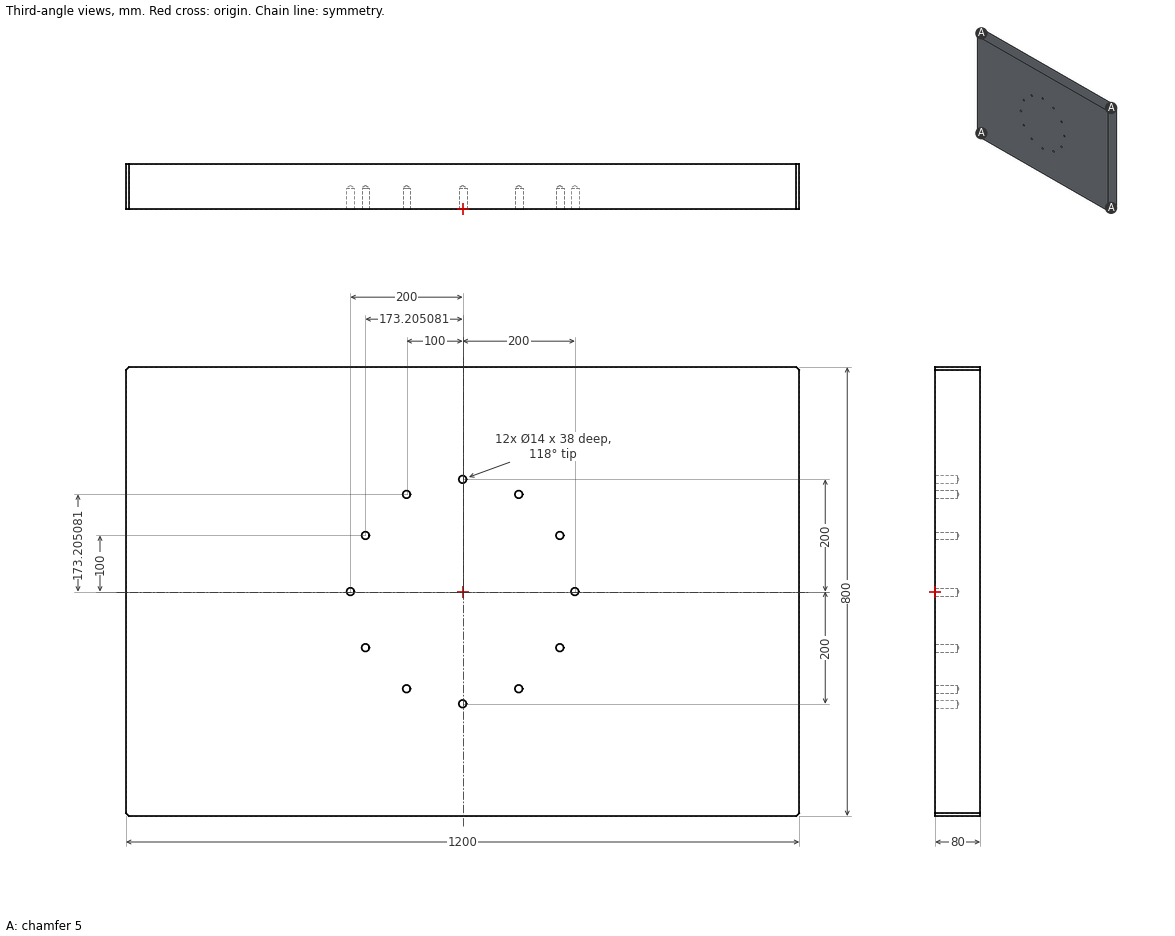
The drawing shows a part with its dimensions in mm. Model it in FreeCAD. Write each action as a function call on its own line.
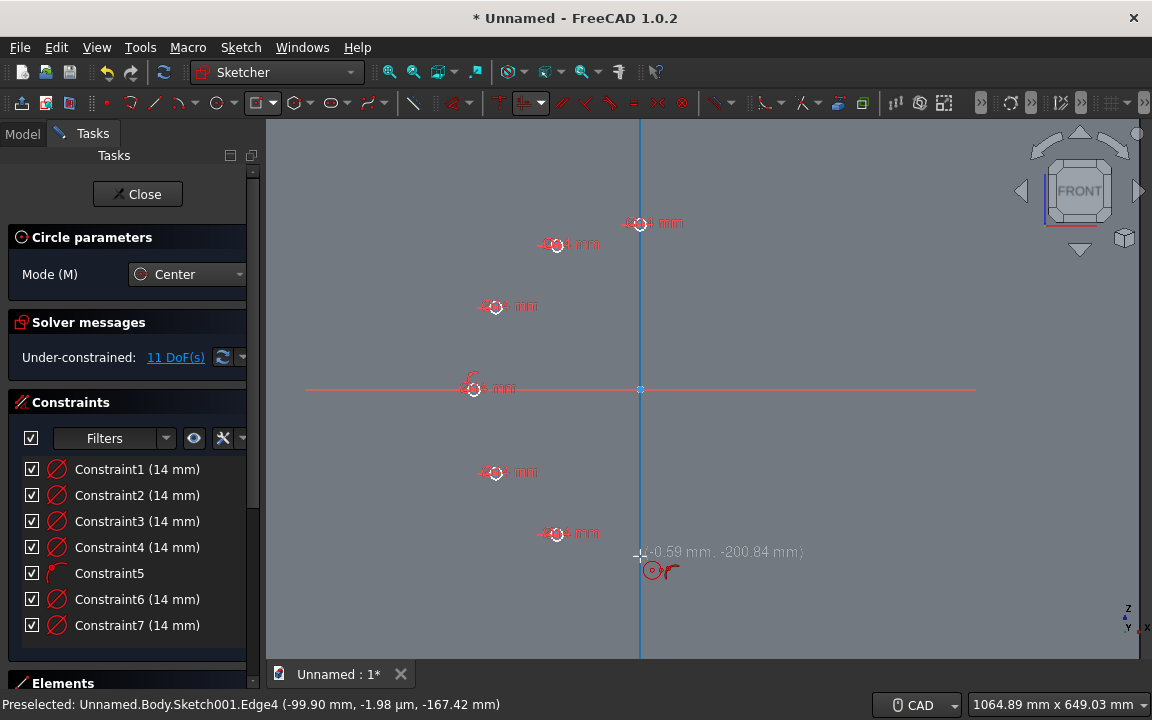
click(640, 556)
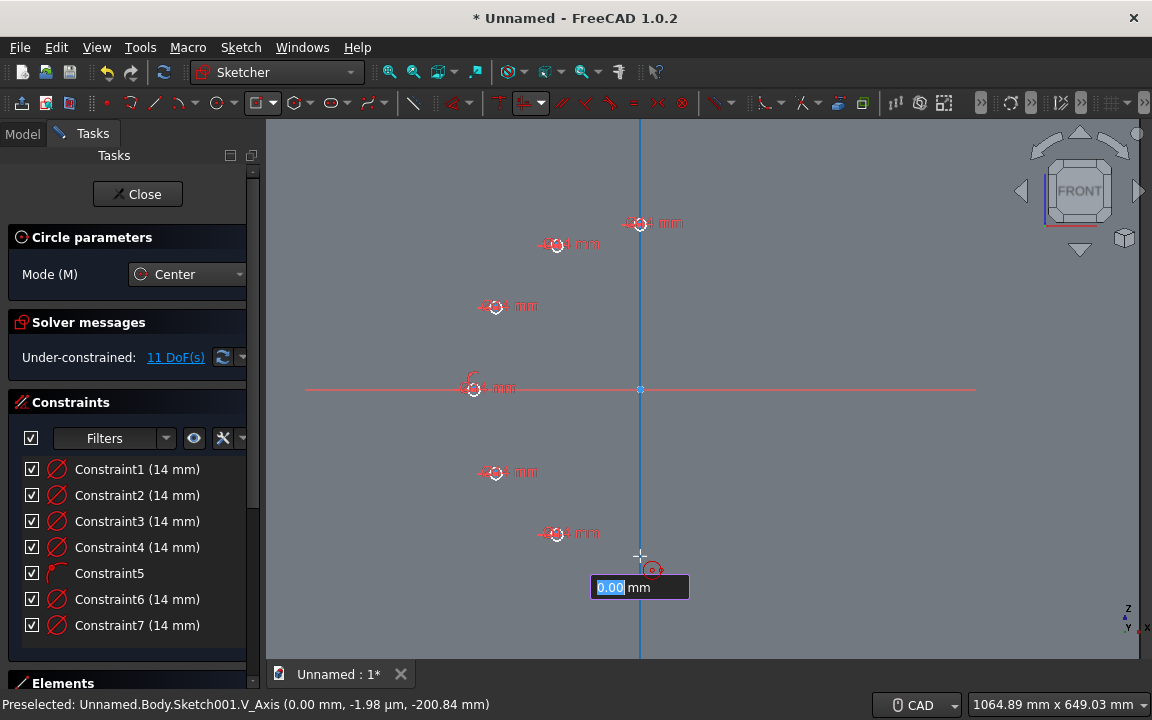
scroll(646, 554, up, 6)
move(645, 553)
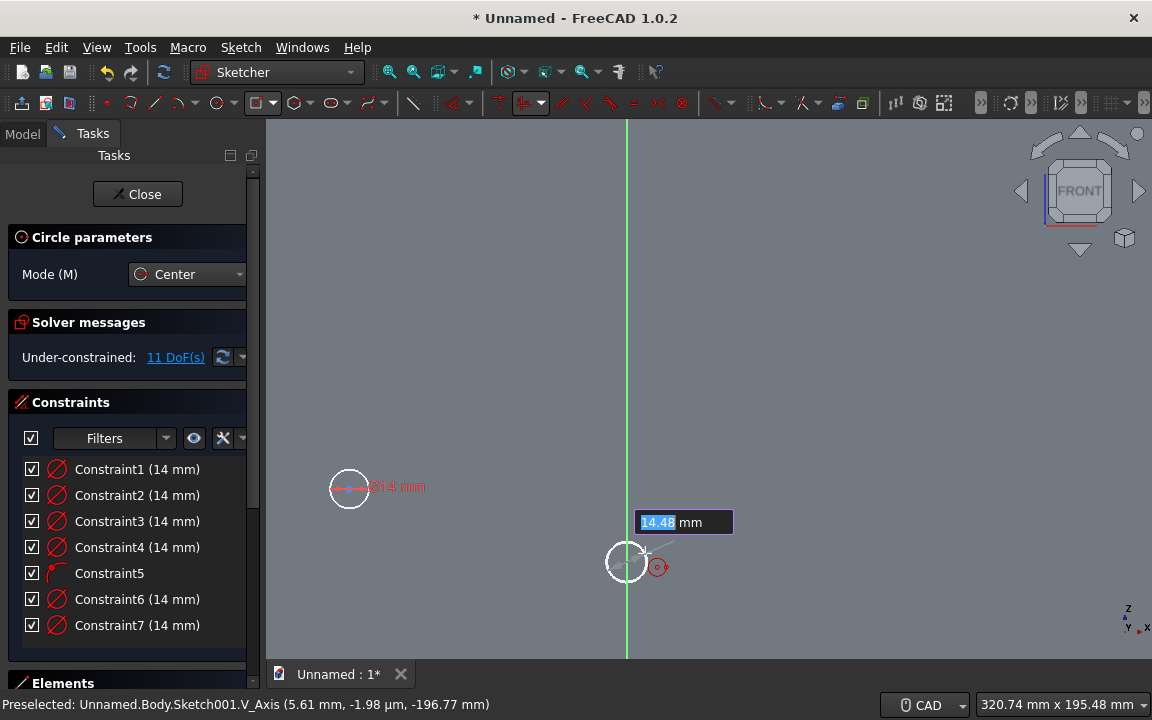
text(14)
key(Return)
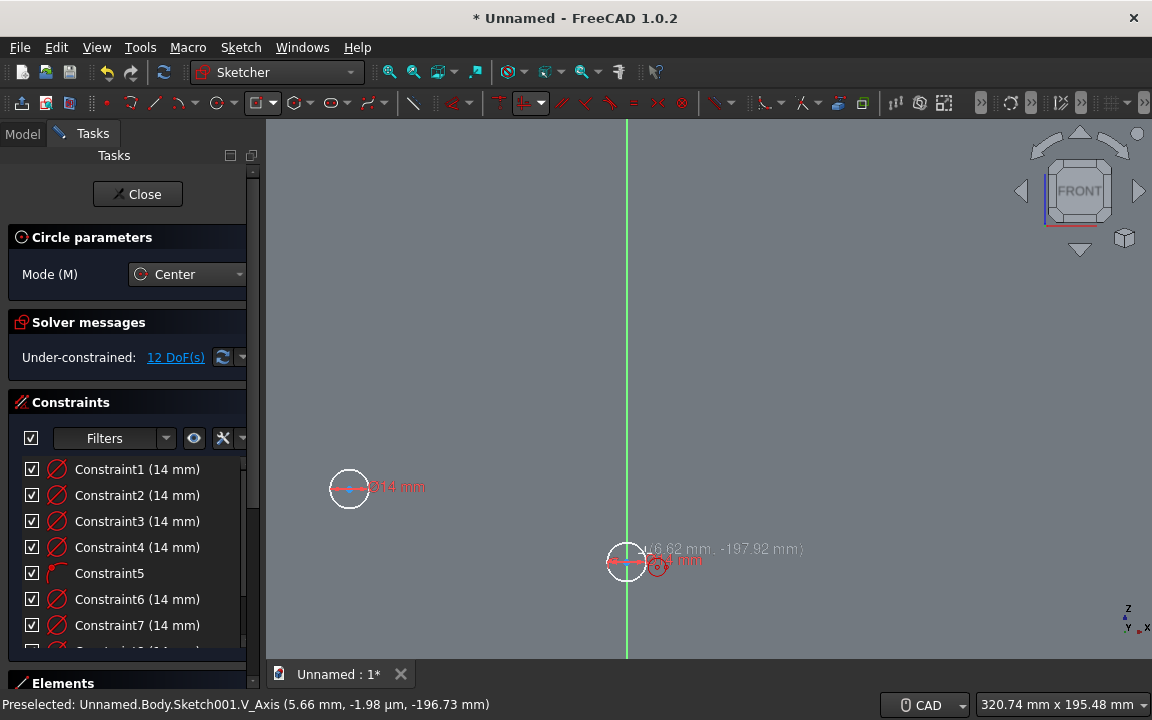
click(903, 486)
move(917, 472)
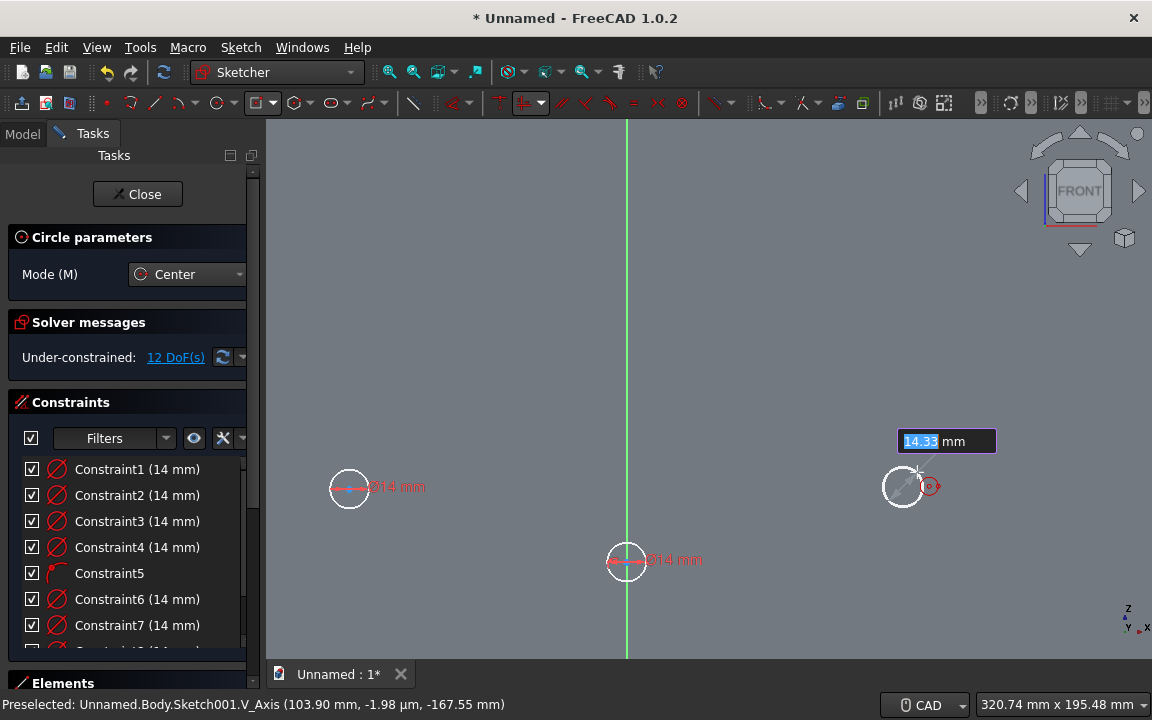
text(14)
key(Return)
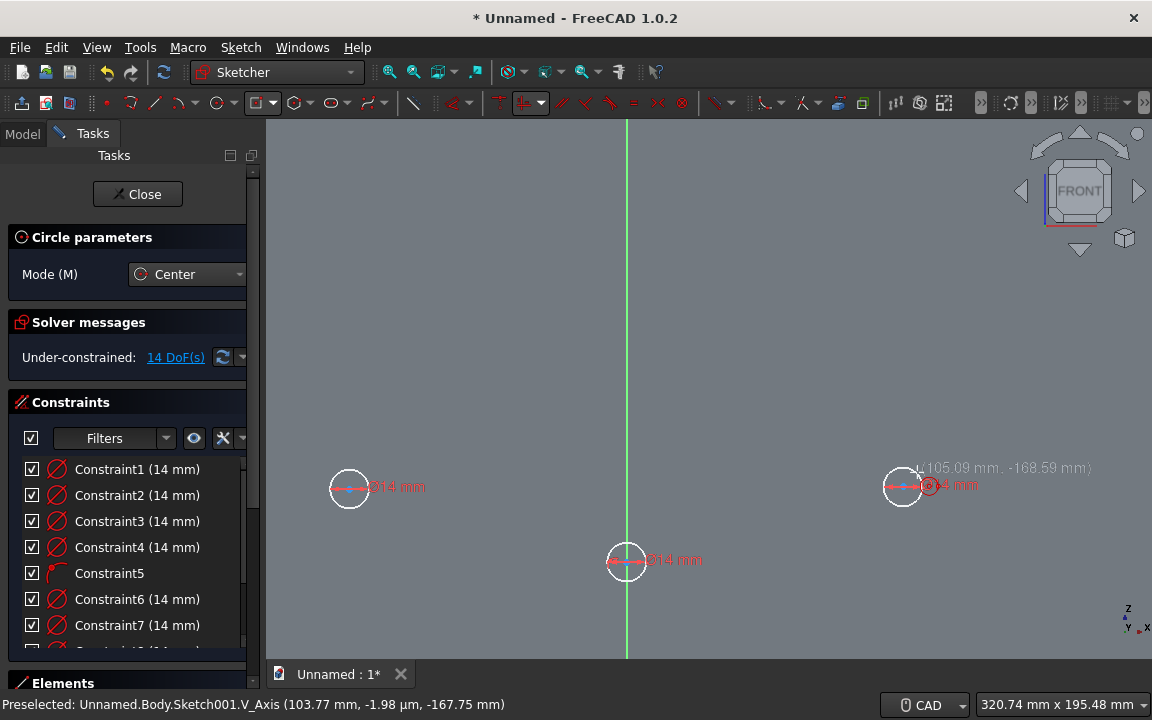
scroll(646, 554, down, 6)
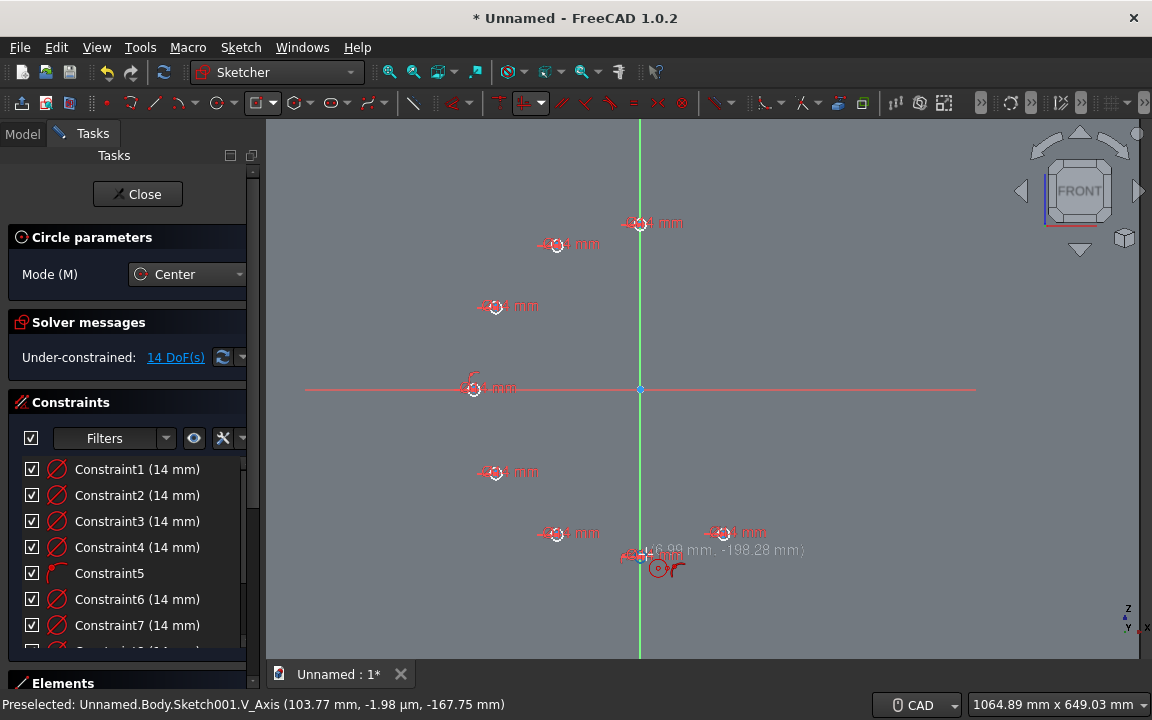
scroll(785, 473, up, 7)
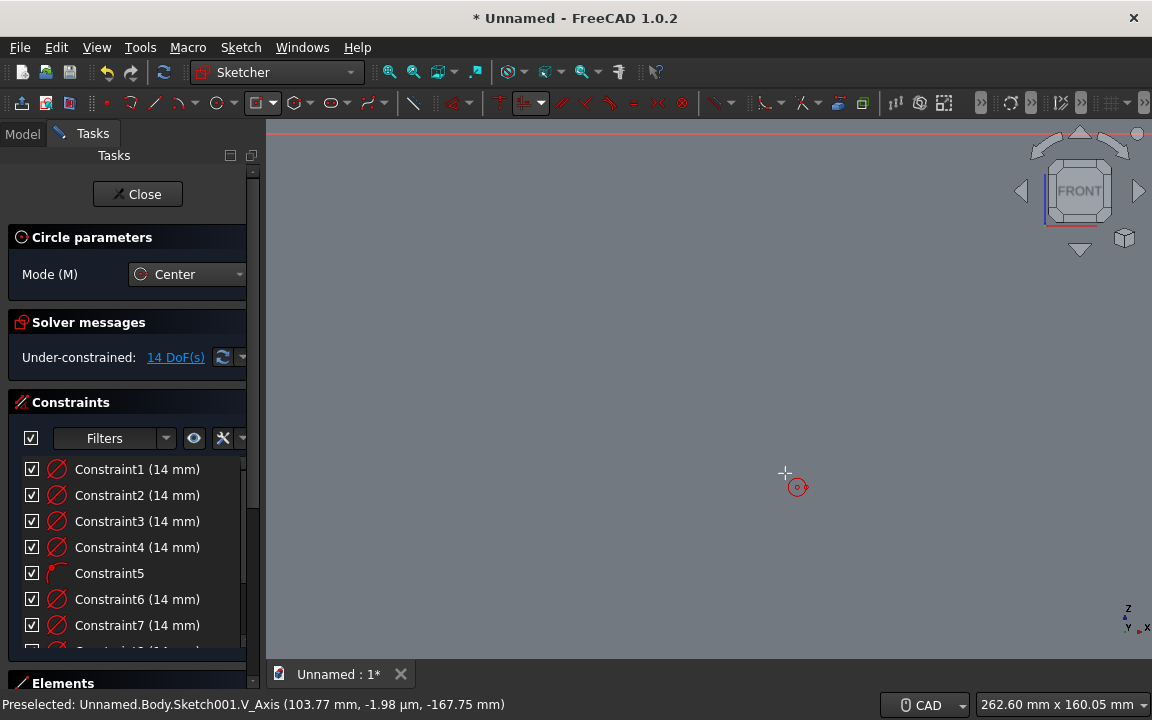
scroll(786, 472, down, 7)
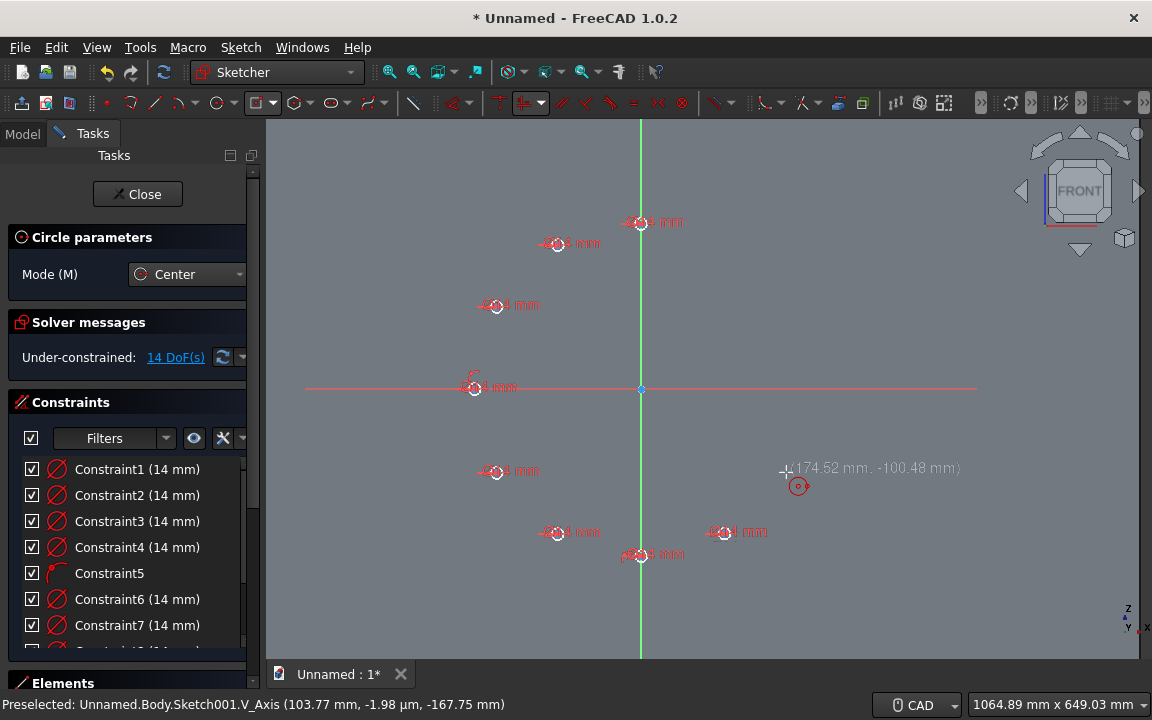
click(785, 472)
move(789, 468)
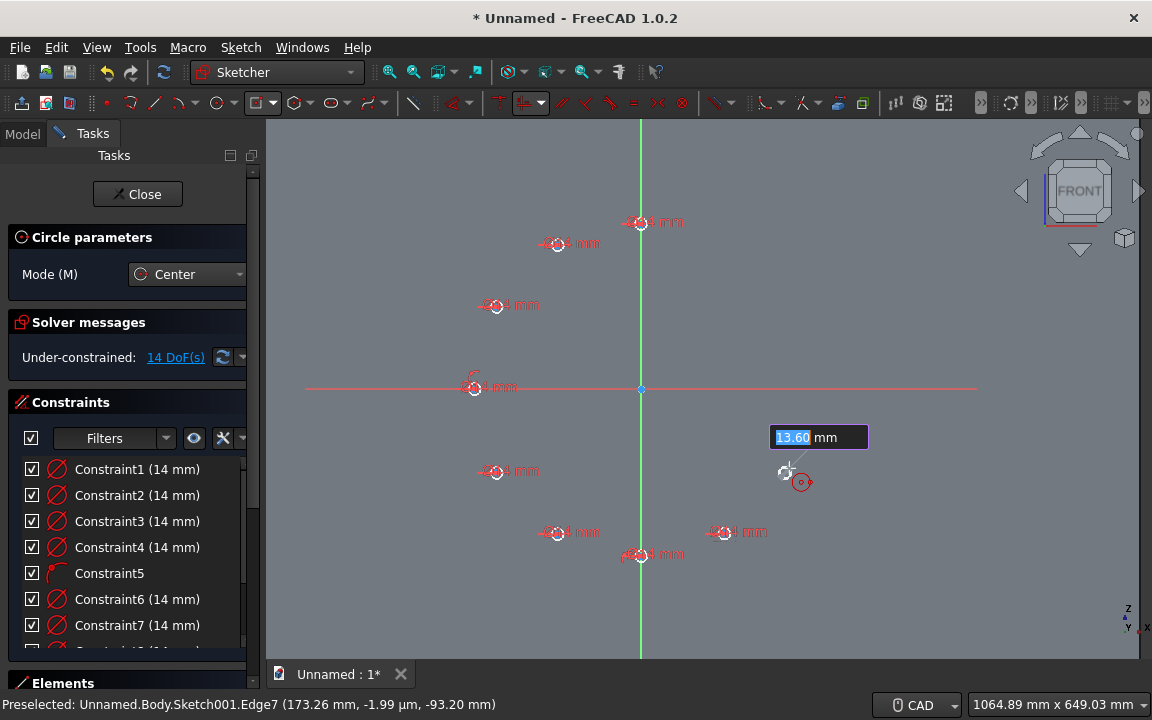
text(14)
key(Return)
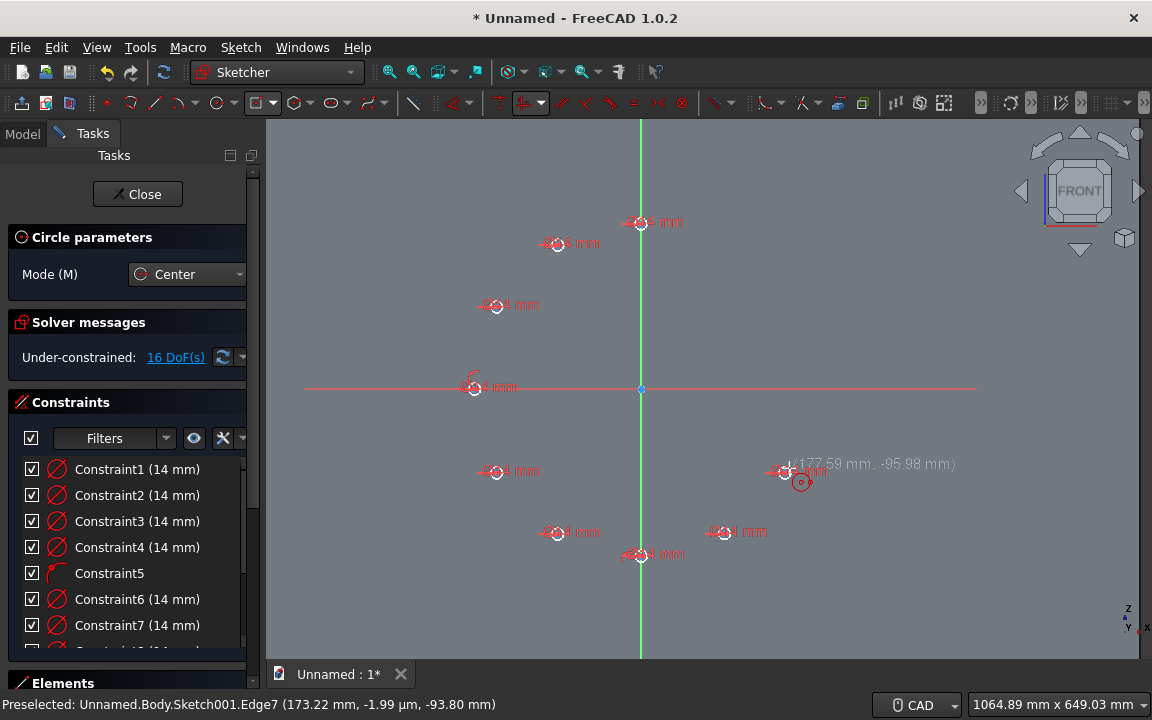
scroll(808, 389, up, 7)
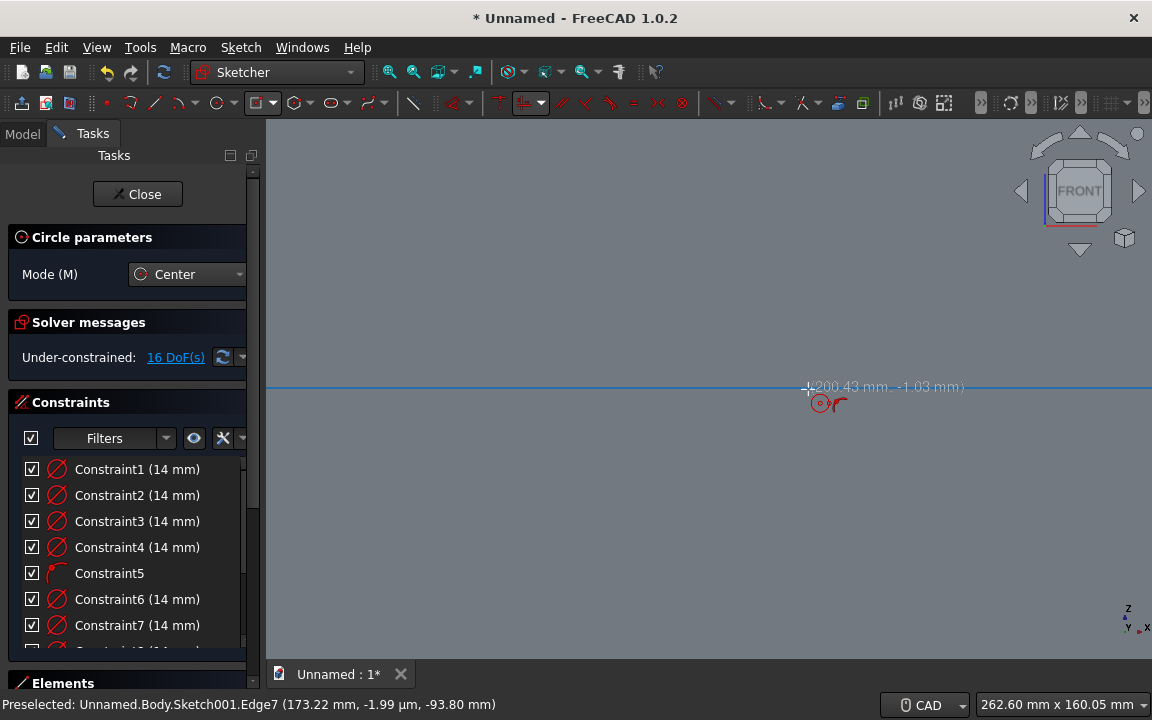
scroll(808, 389, down, 7)